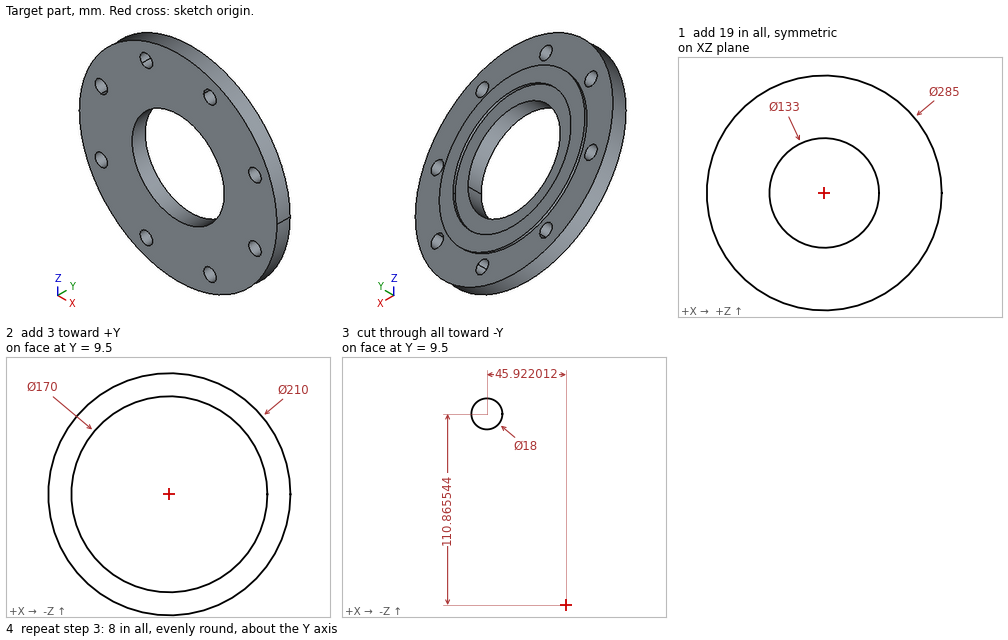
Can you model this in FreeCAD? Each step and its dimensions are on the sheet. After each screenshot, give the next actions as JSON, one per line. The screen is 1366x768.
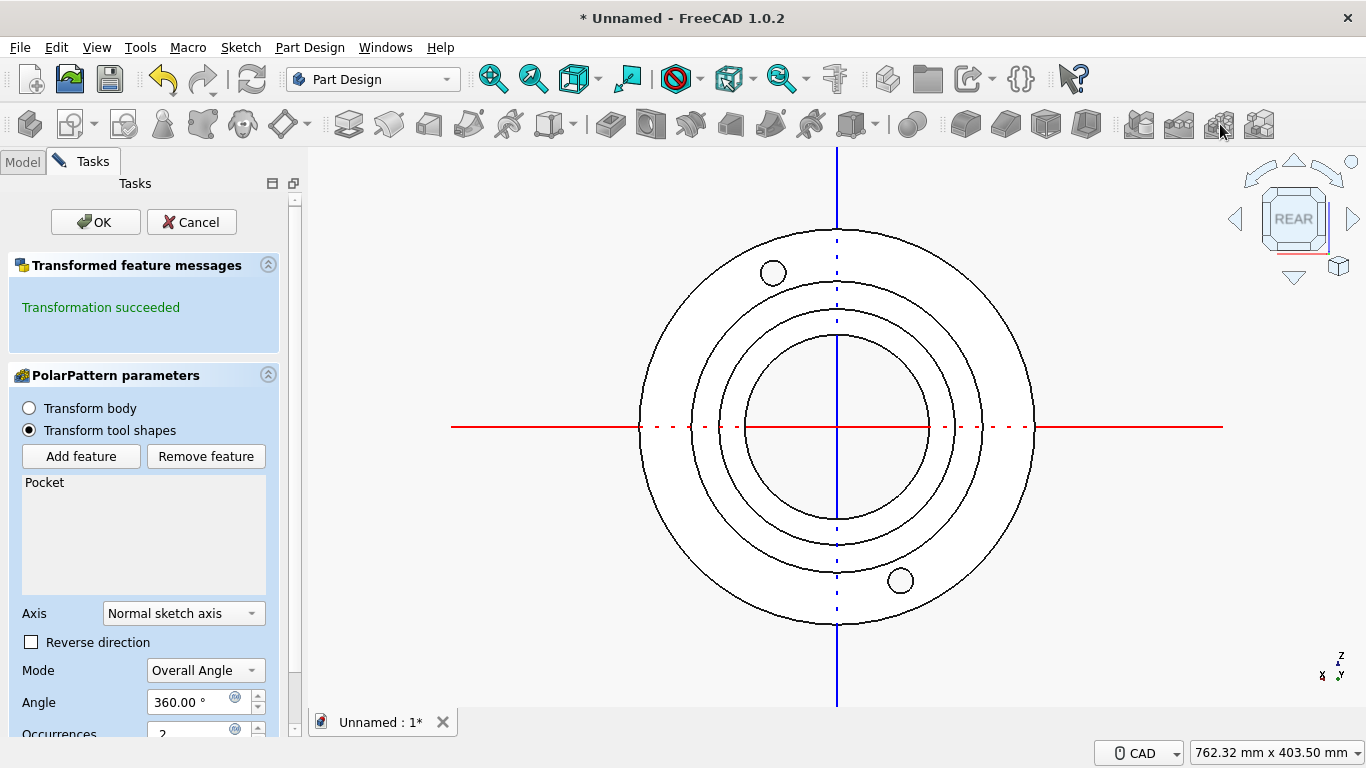
{"action": "left_click", "coordinate": [184, 614]}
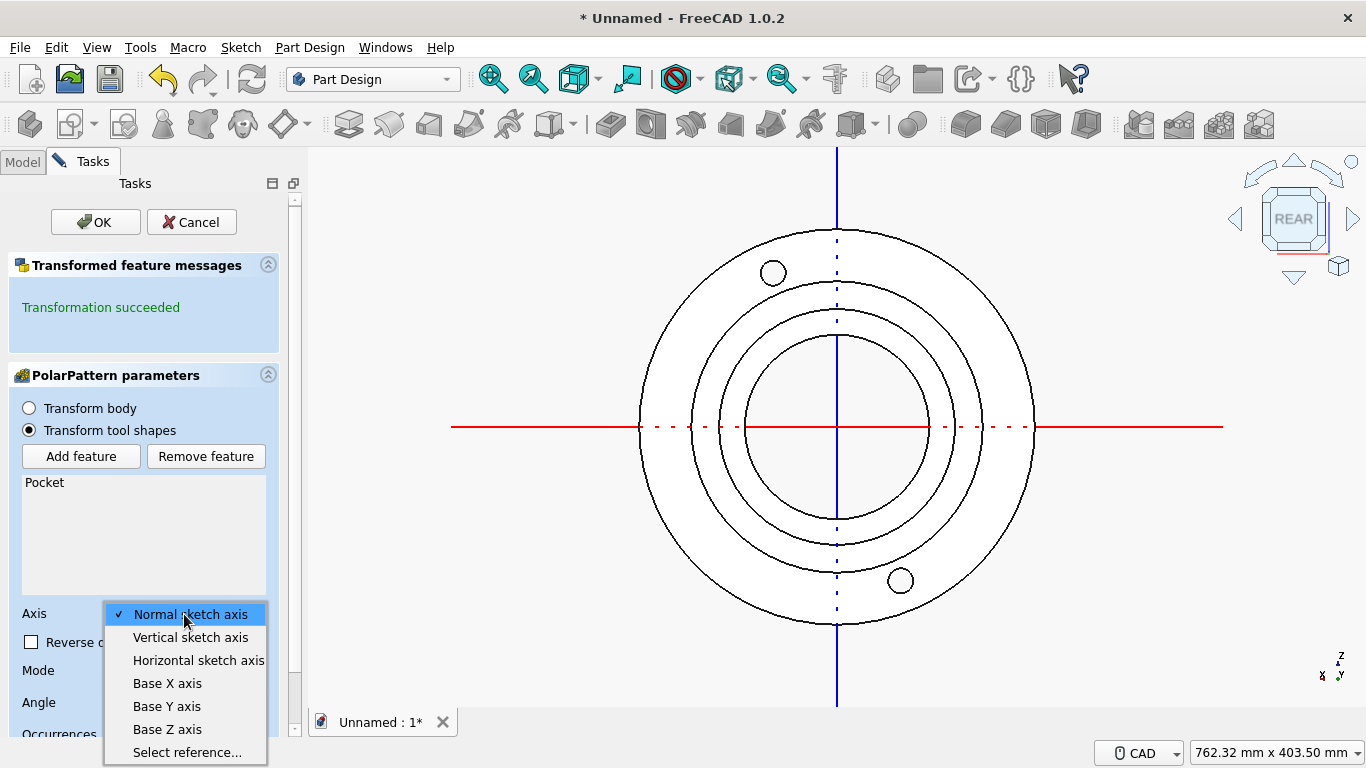
{"action": "left_click", "coordinate": [184, 706]}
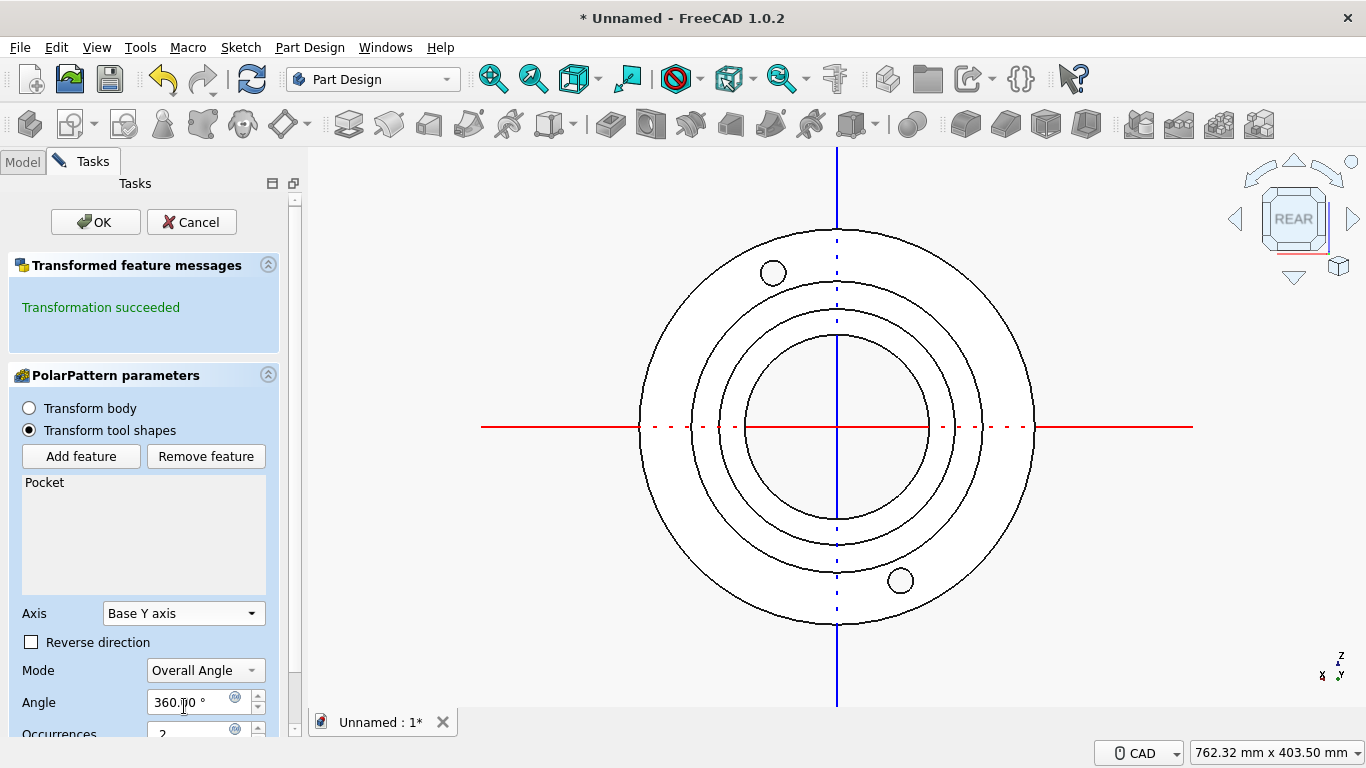
{"action": "scroll", "coordinate": [295, 464], "scroll_direction": "down", "scroll_amount": 2}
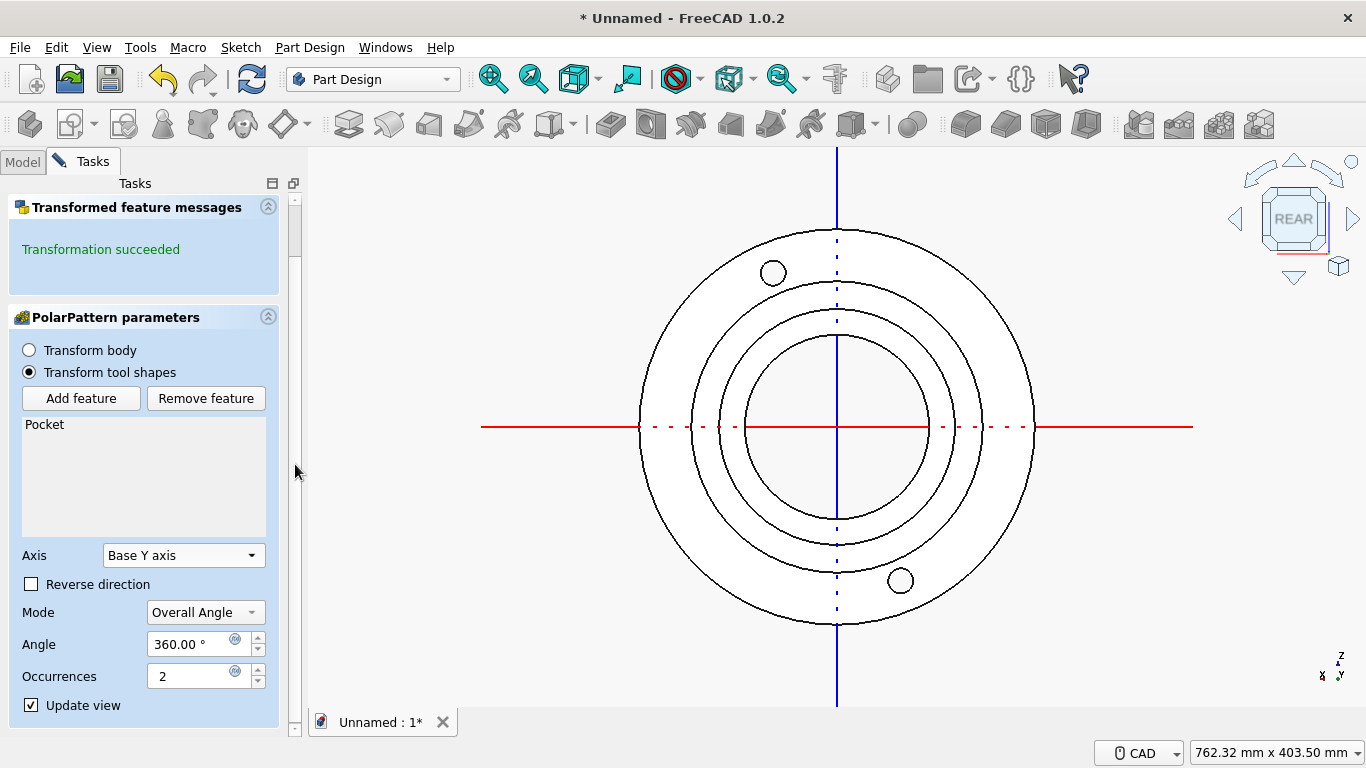
{"action": "triple_click", "coordinate": [198, 676]}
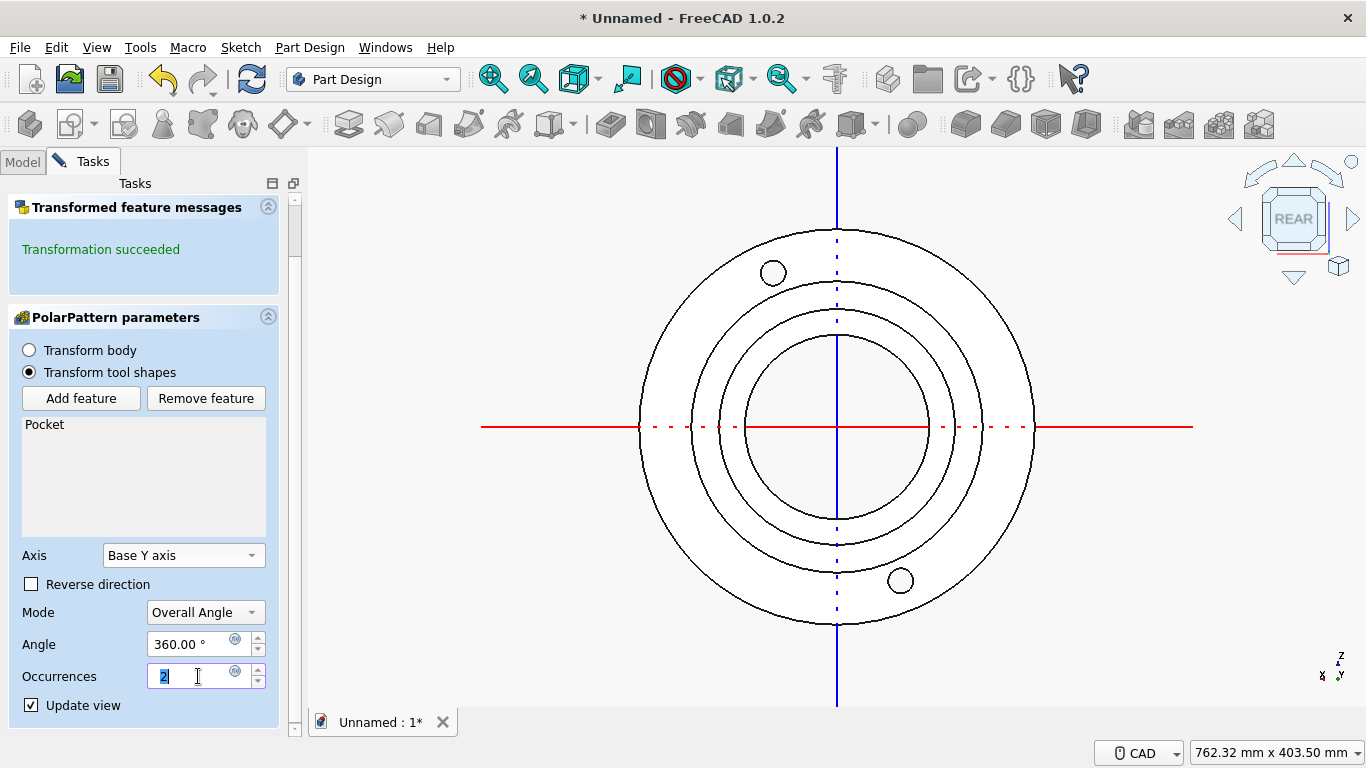
{"action": "type", "text": "8"}
{"action": "key", "text": "Tab"}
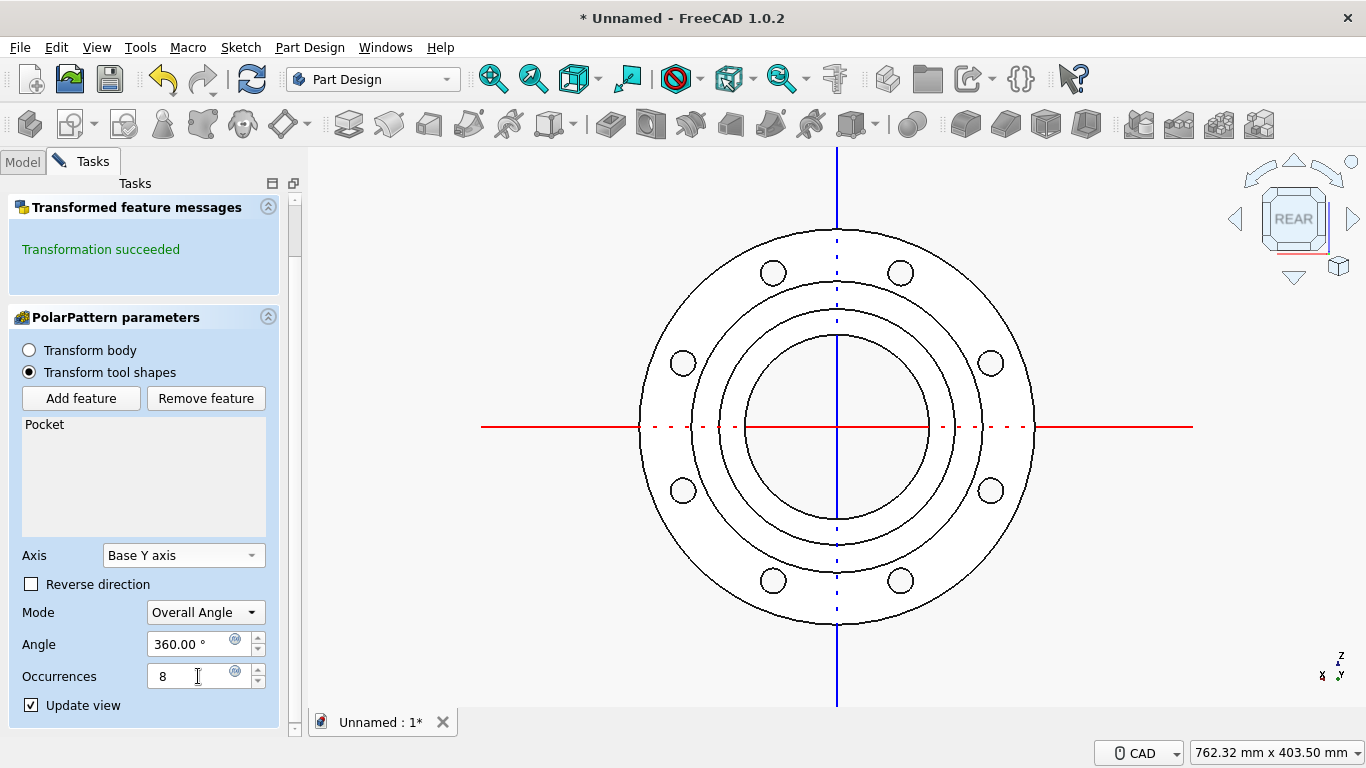
{"action": "scroll", "coordinate": [295, 464], "scroll_direction": "up", "scroll_amount": 2}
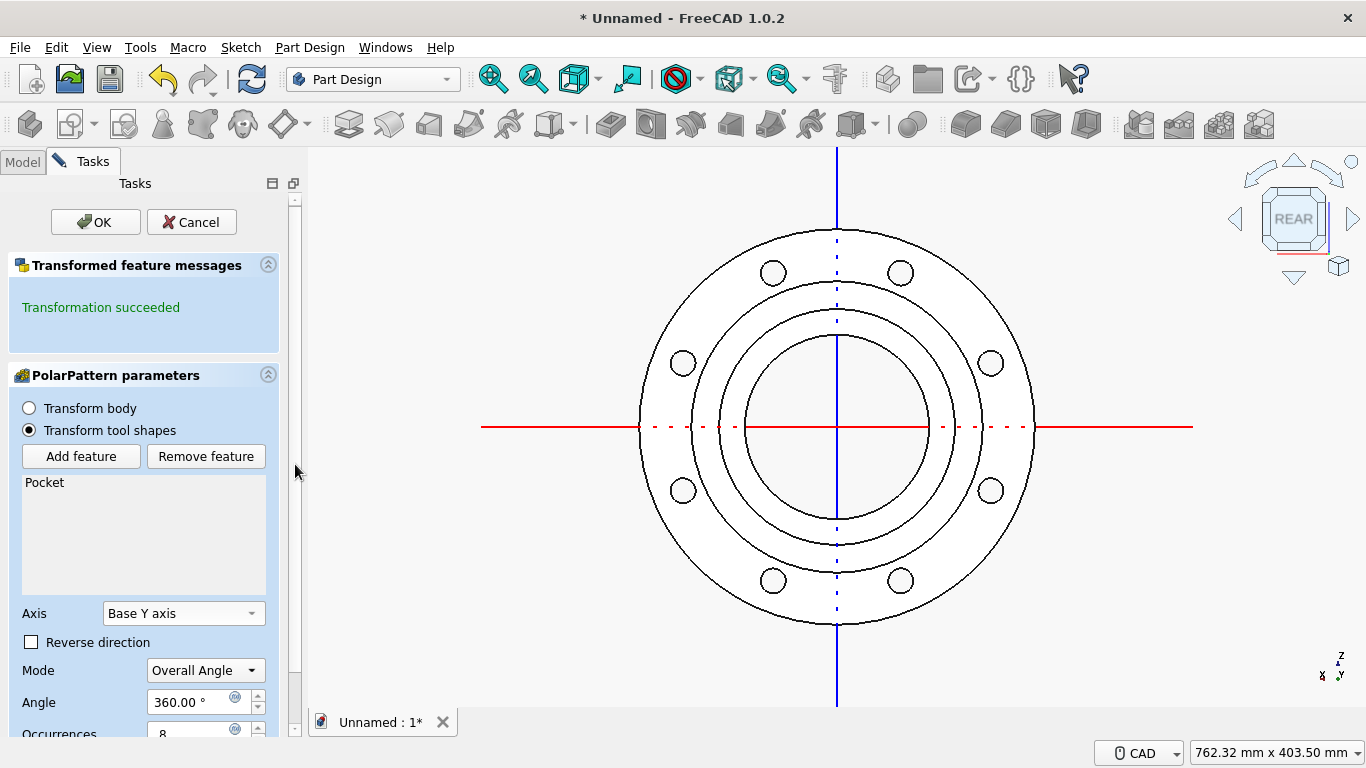
{"action": "left_click", "coordinate": [96, 222]}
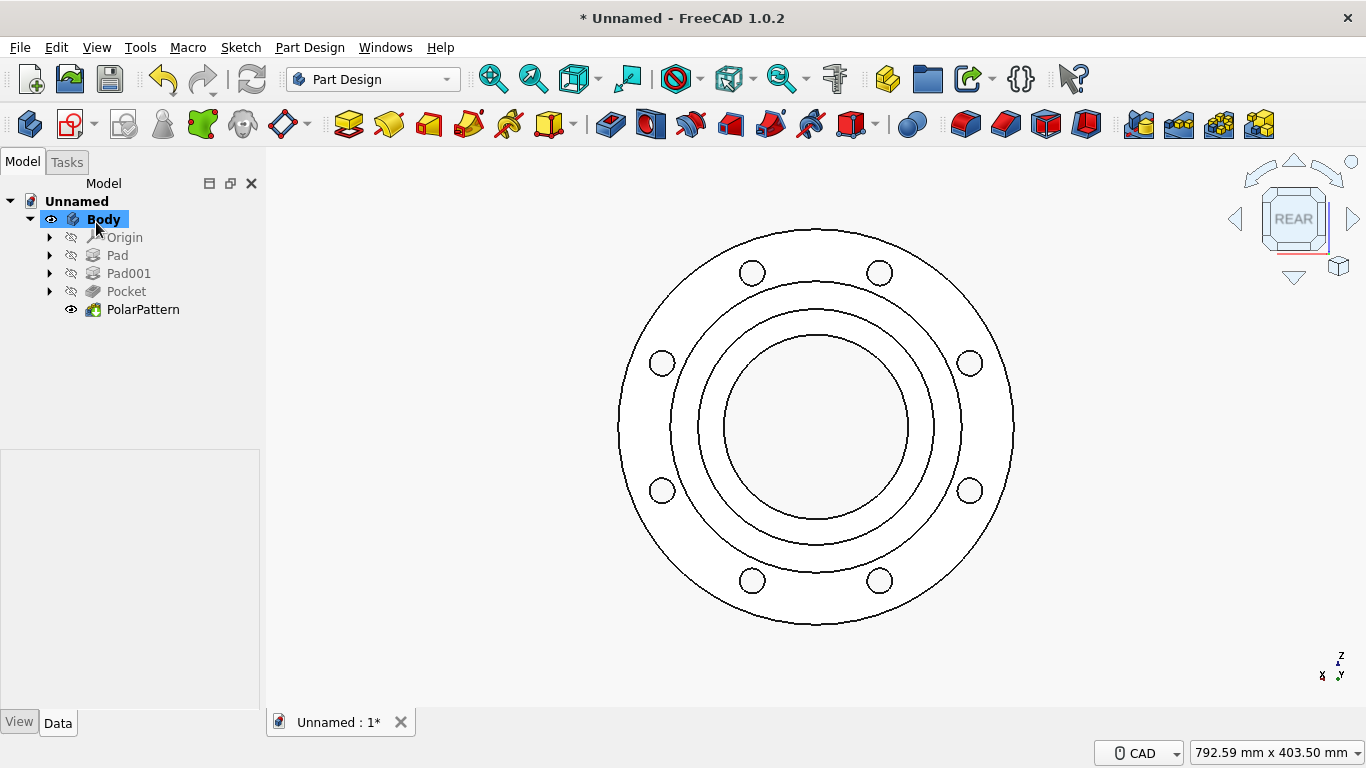
{"action": "key", "text": "0"}